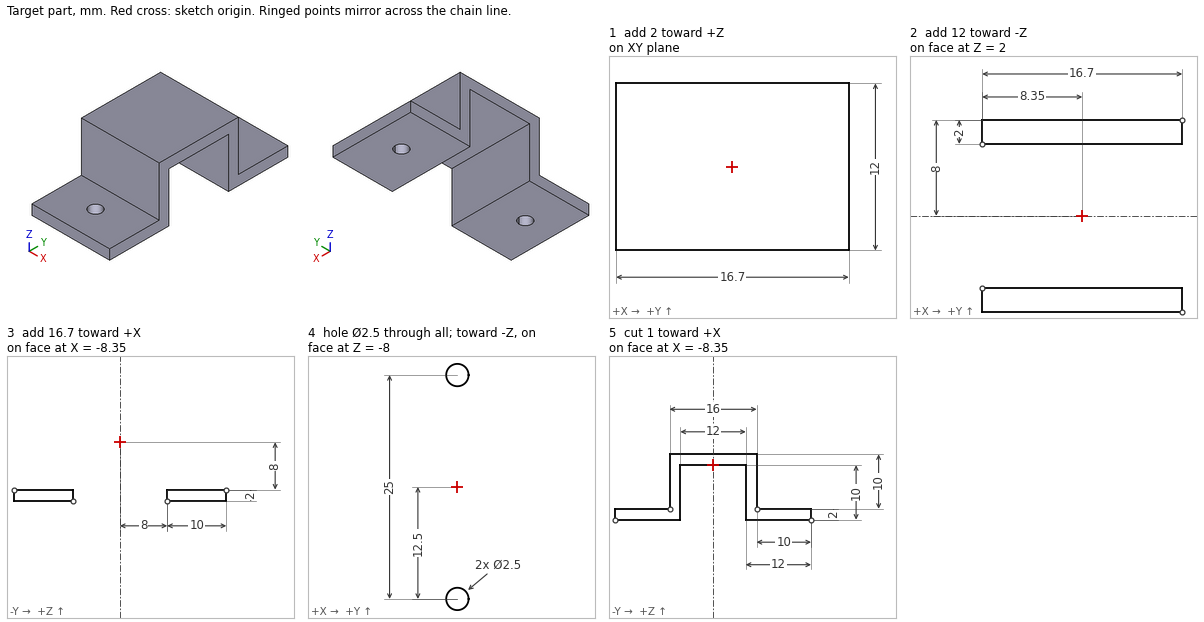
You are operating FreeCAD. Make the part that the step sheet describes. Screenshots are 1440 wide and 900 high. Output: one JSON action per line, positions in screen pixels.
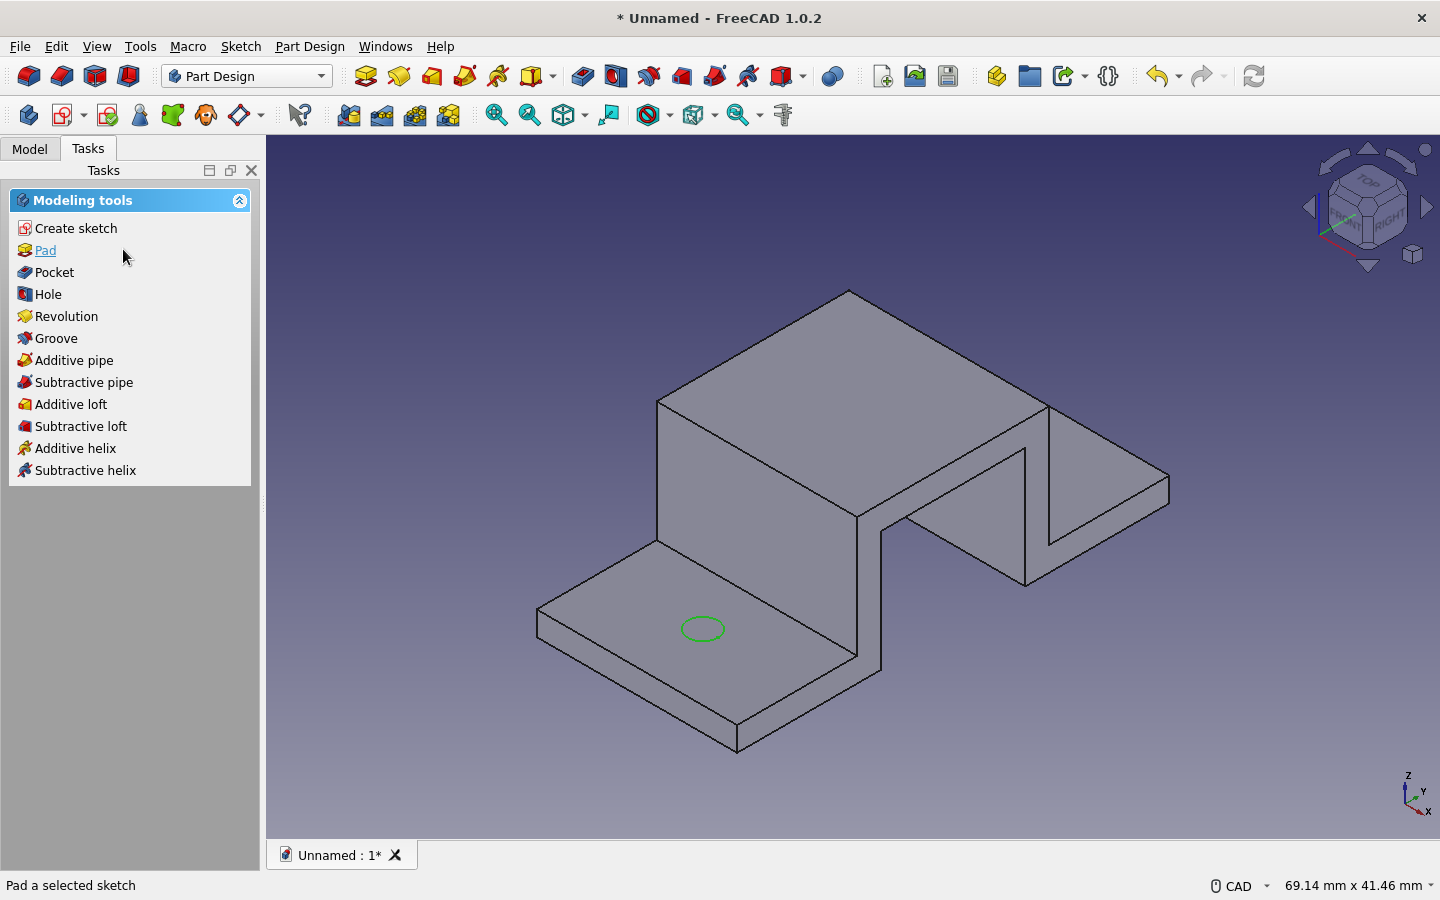
{"action": "left_click", "coordinate": [616, 76]}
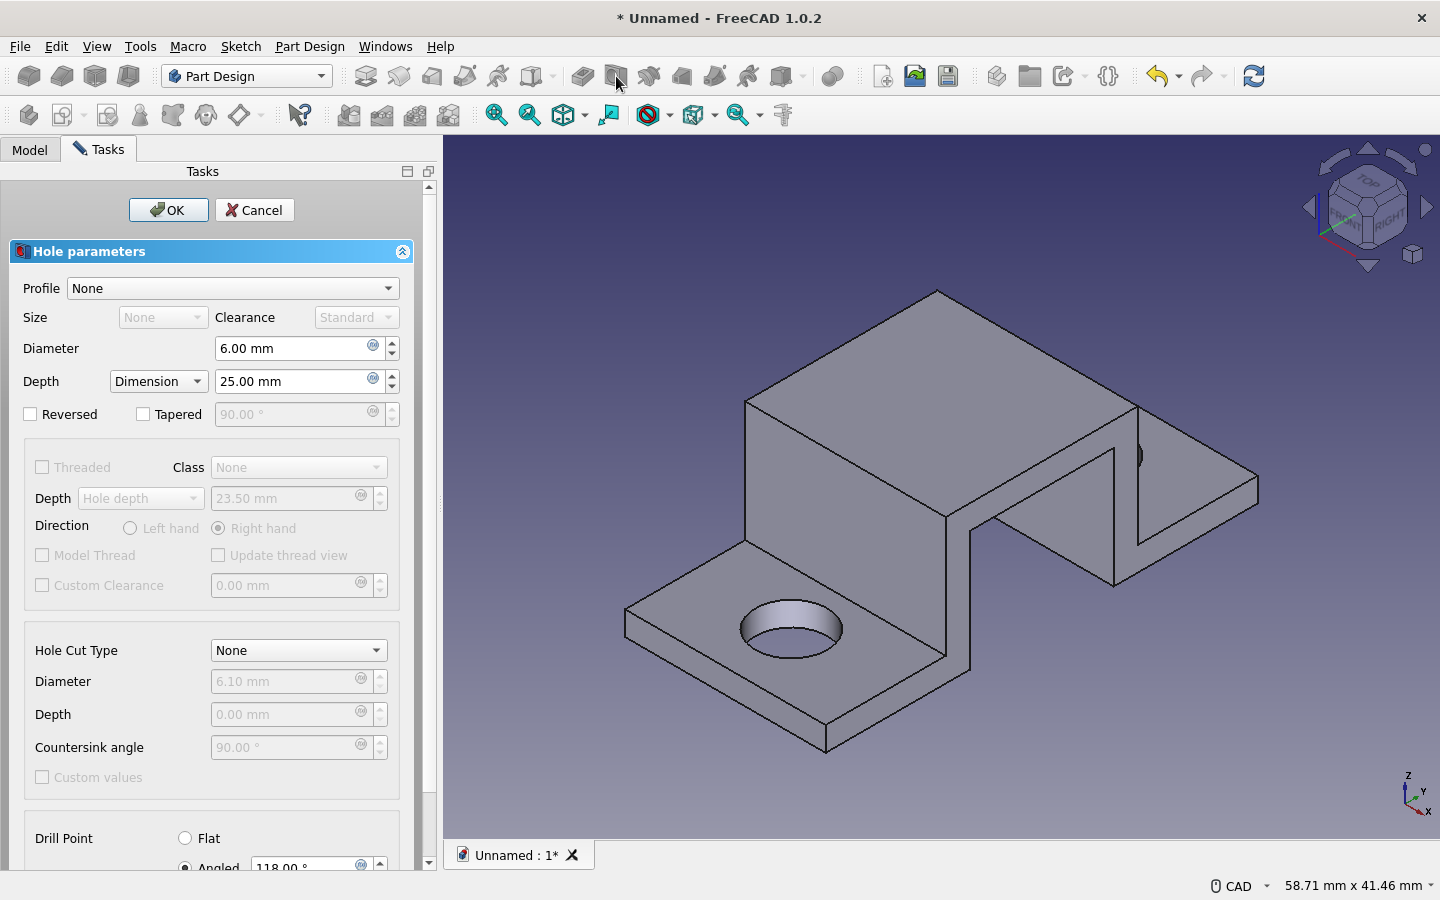
{"action": "triple_click", "coordinate": [300, 348]}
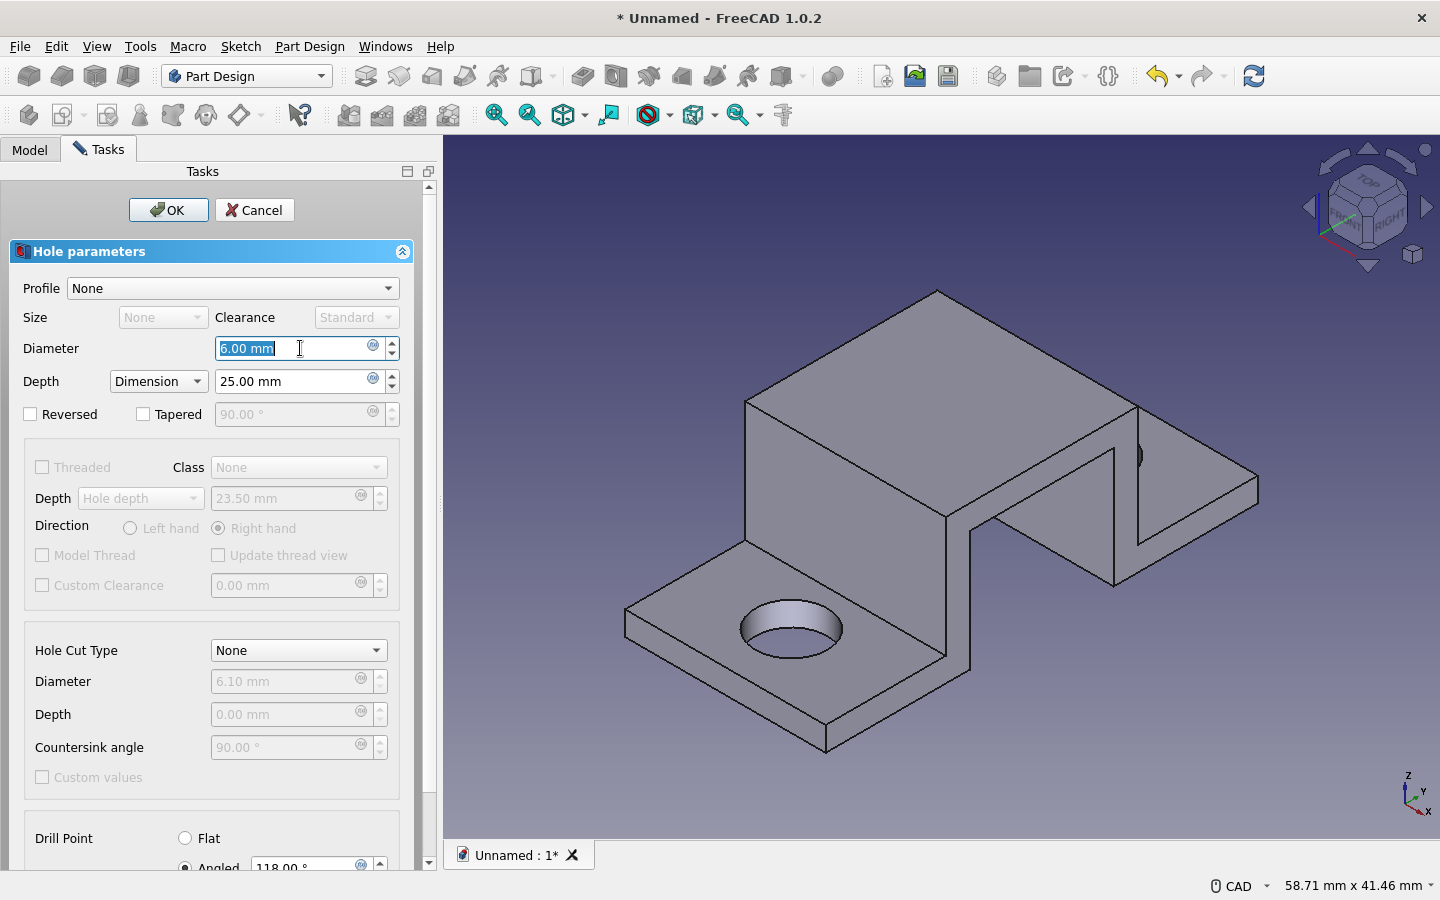
{"action": "type", "text": "2.5"}
{"action": "key", "text": "Tab"}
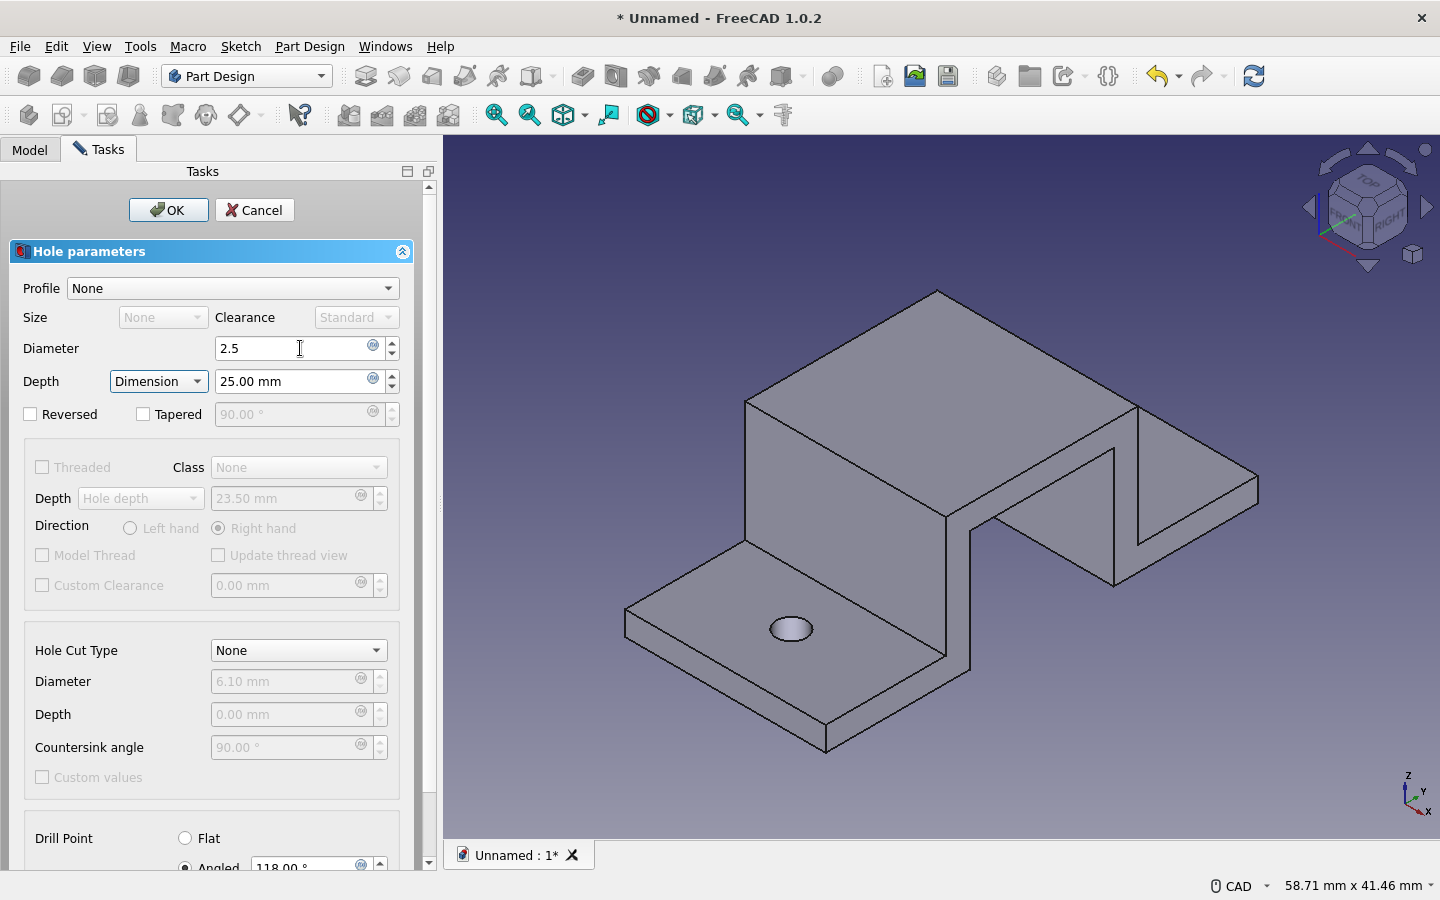
{"action": "left_click", "coordinate": [160, 382]}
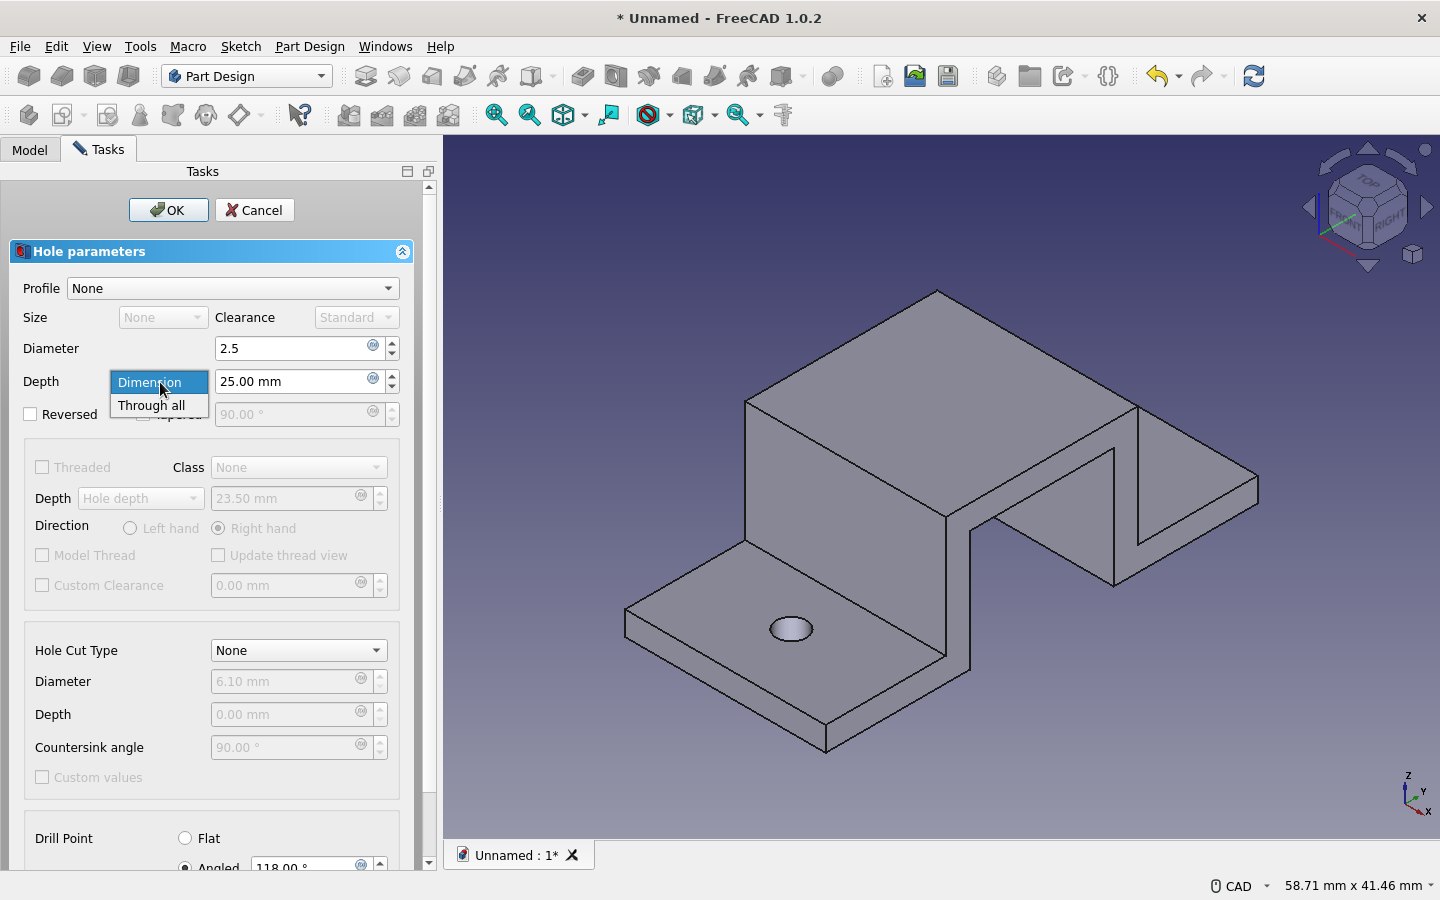
{"action": "left_click", "coordinate": [158, 406]}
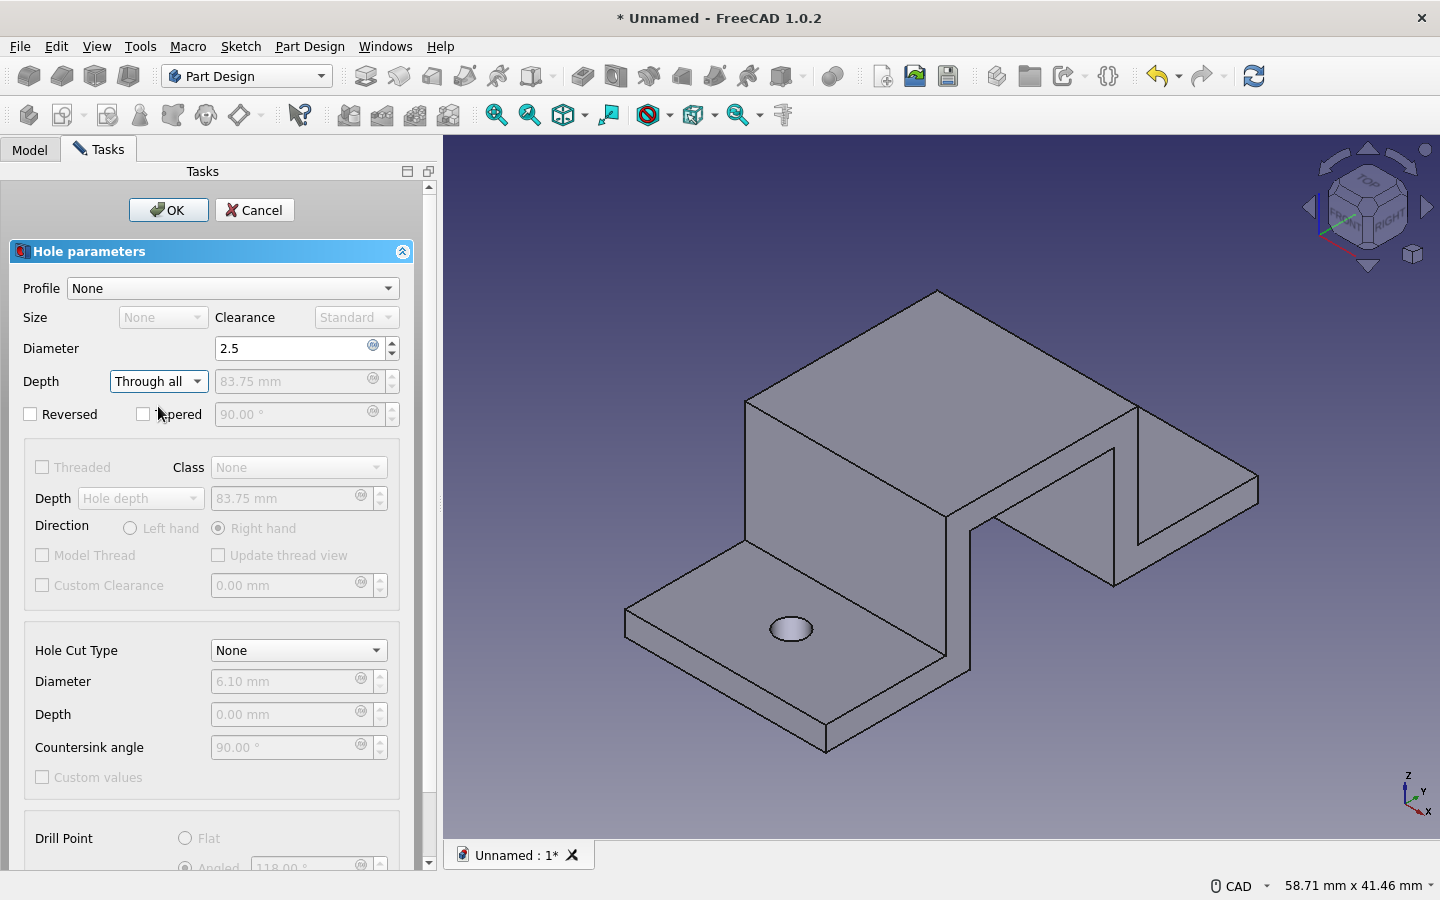
{"action": "left_click", "coordinate": [169, 210]}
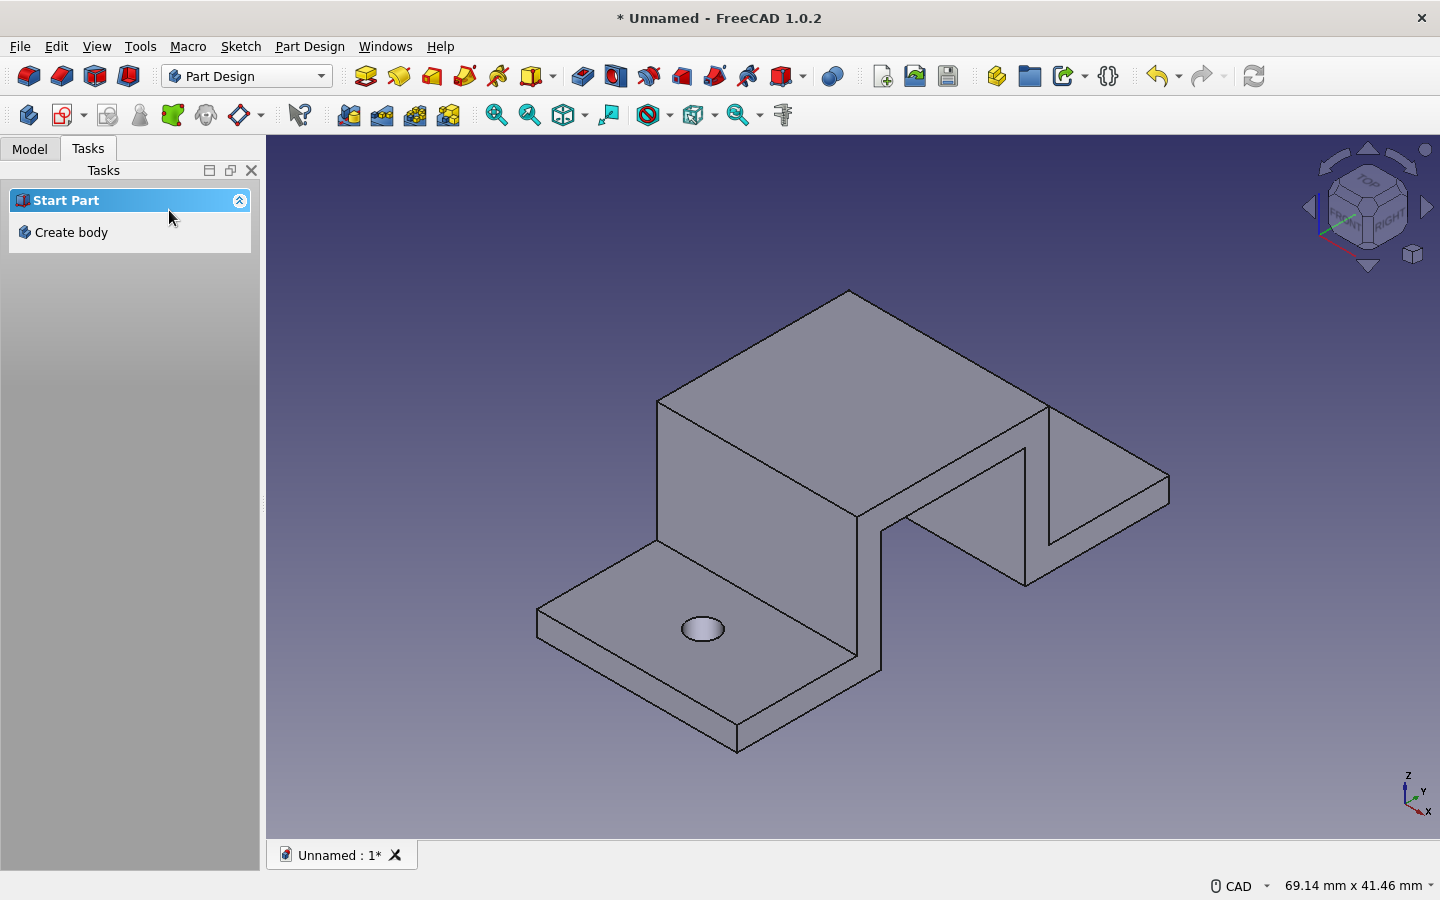
{"action": "key", "text": "6"}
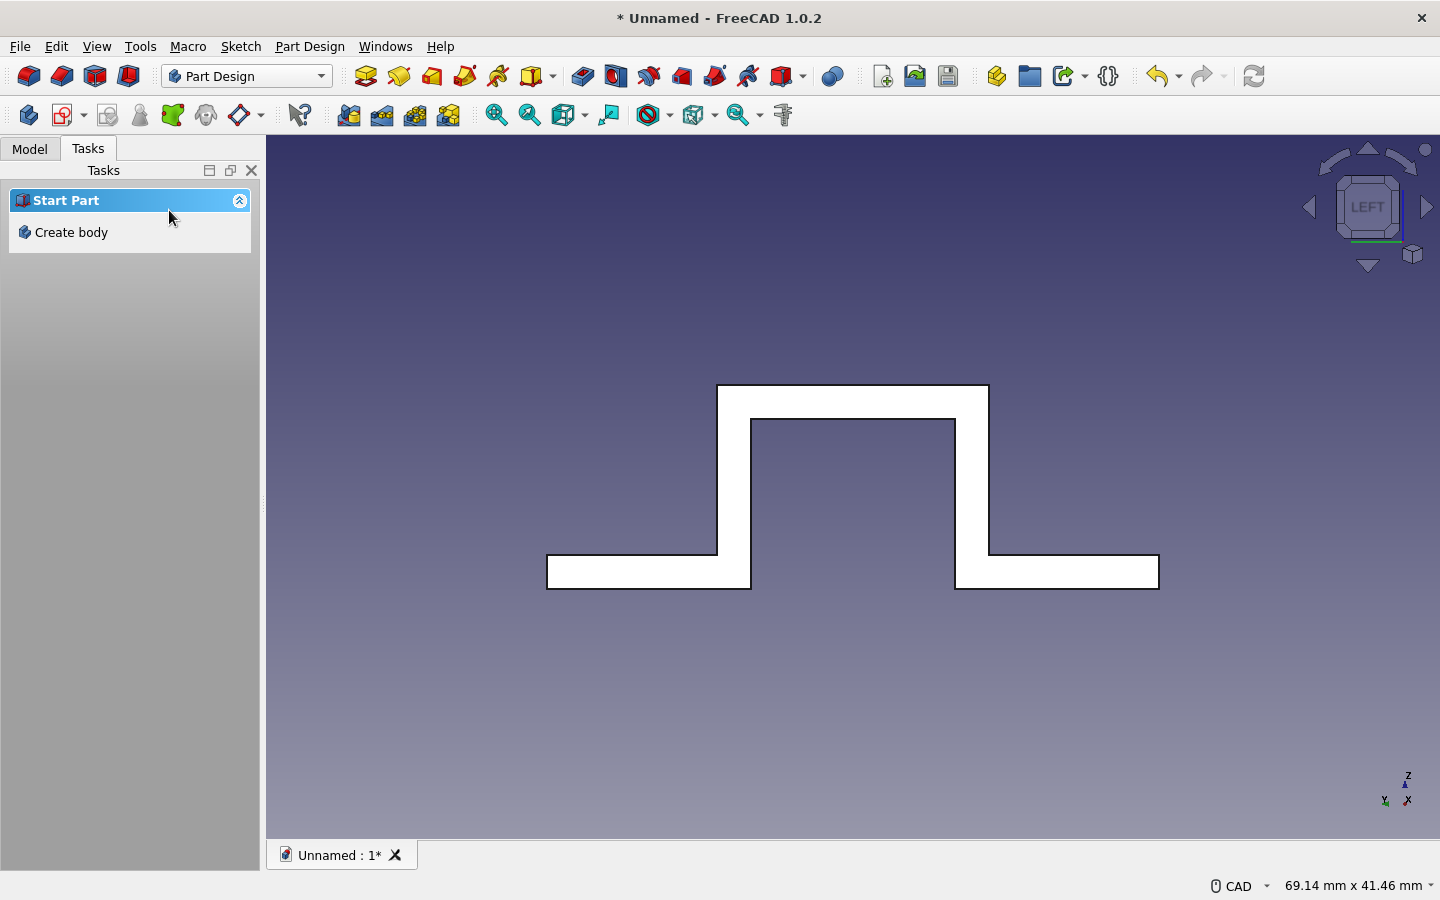
{"action": "left_click", "coordinate": [591, 573]}